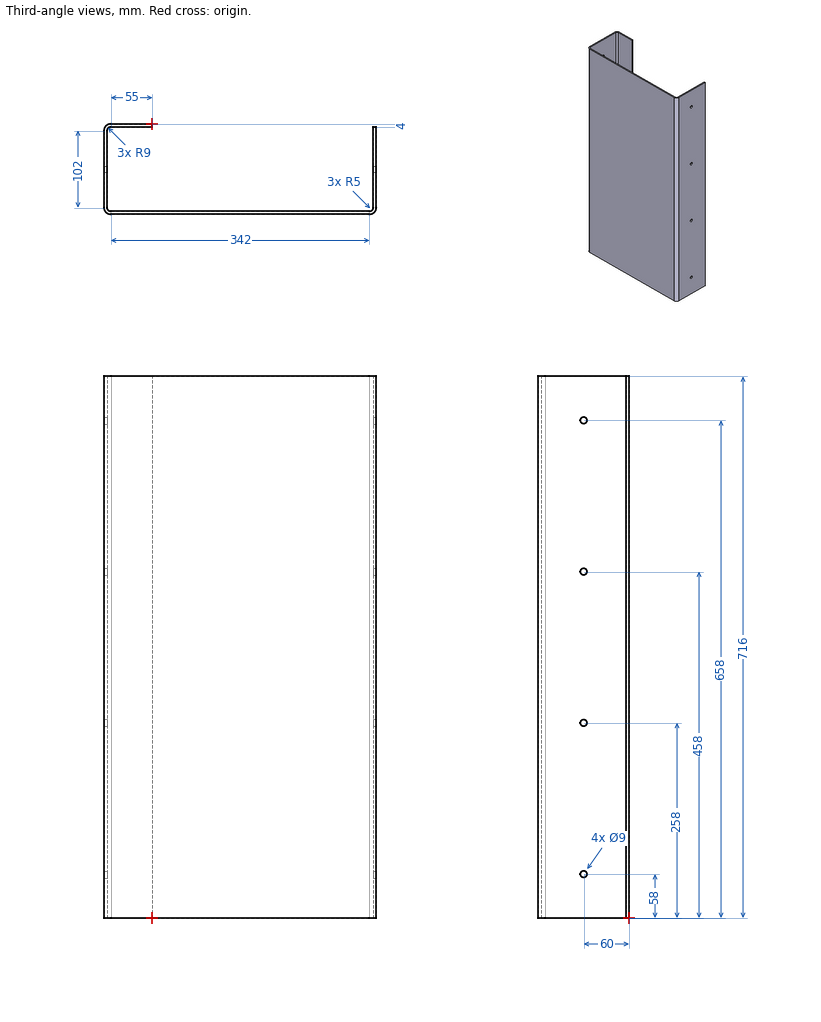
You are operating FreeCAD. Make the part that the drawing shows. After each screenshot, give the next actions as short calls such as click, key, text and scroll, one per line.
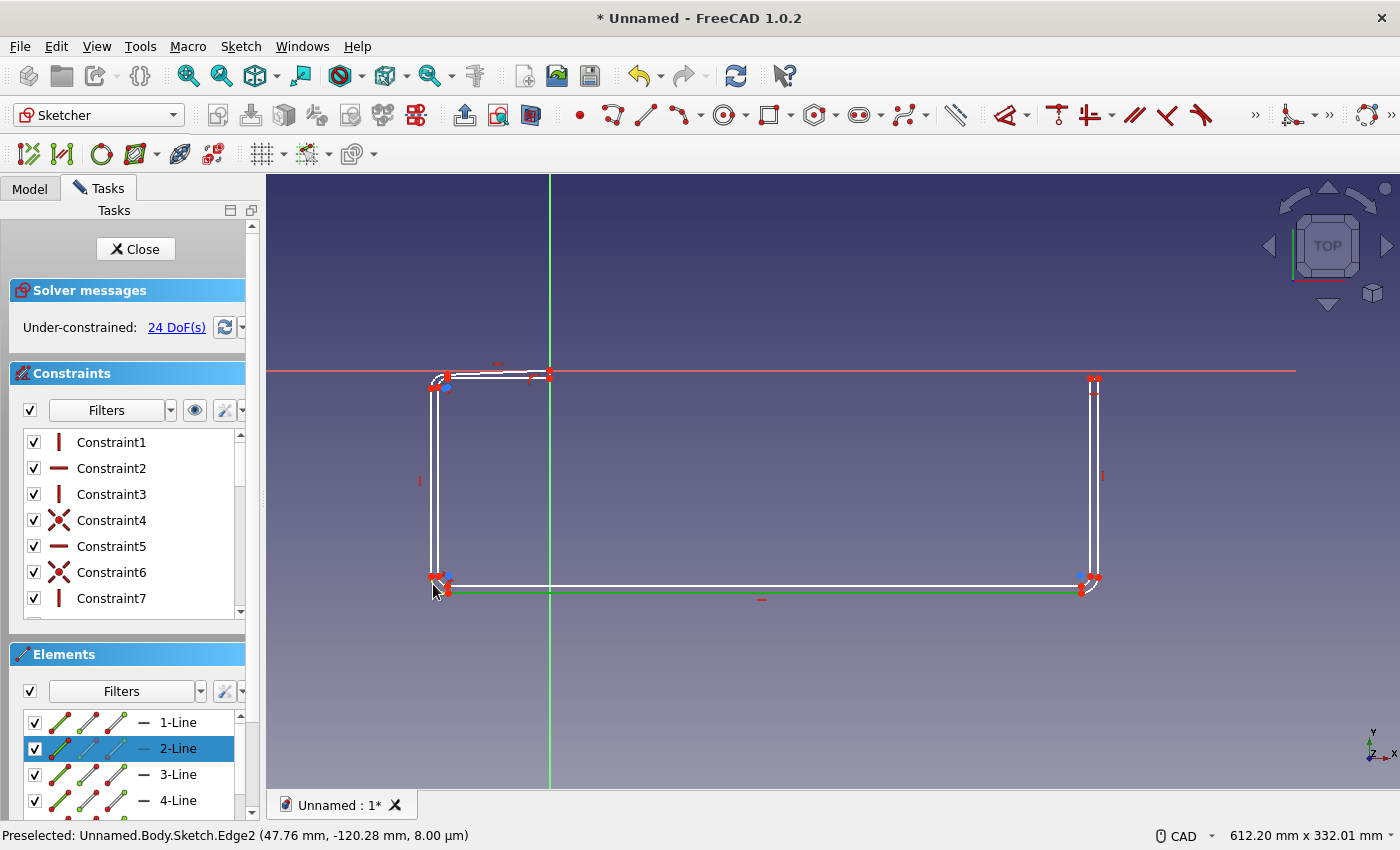
scroll(1088, 591, up, 4)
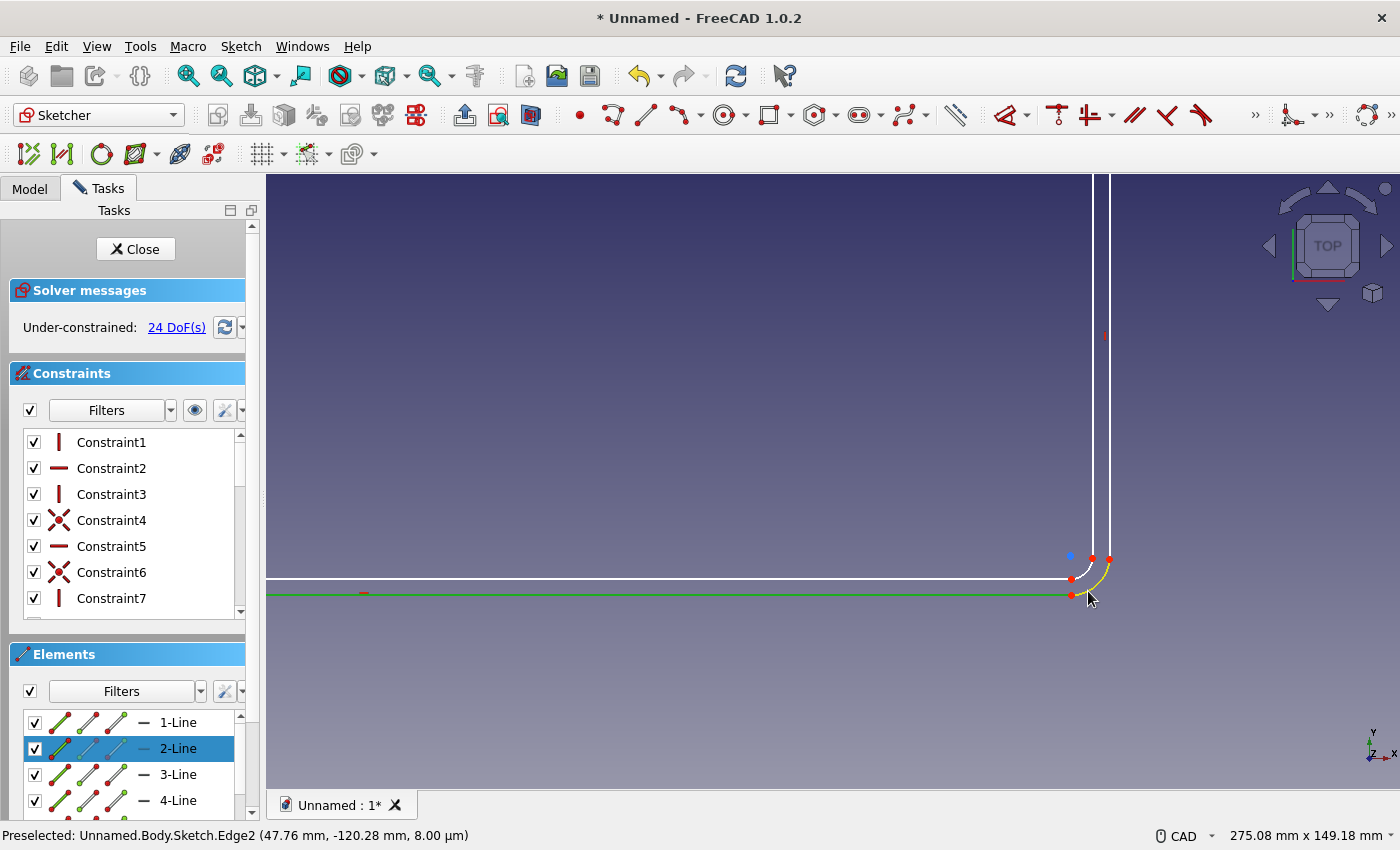
click(1088, 591)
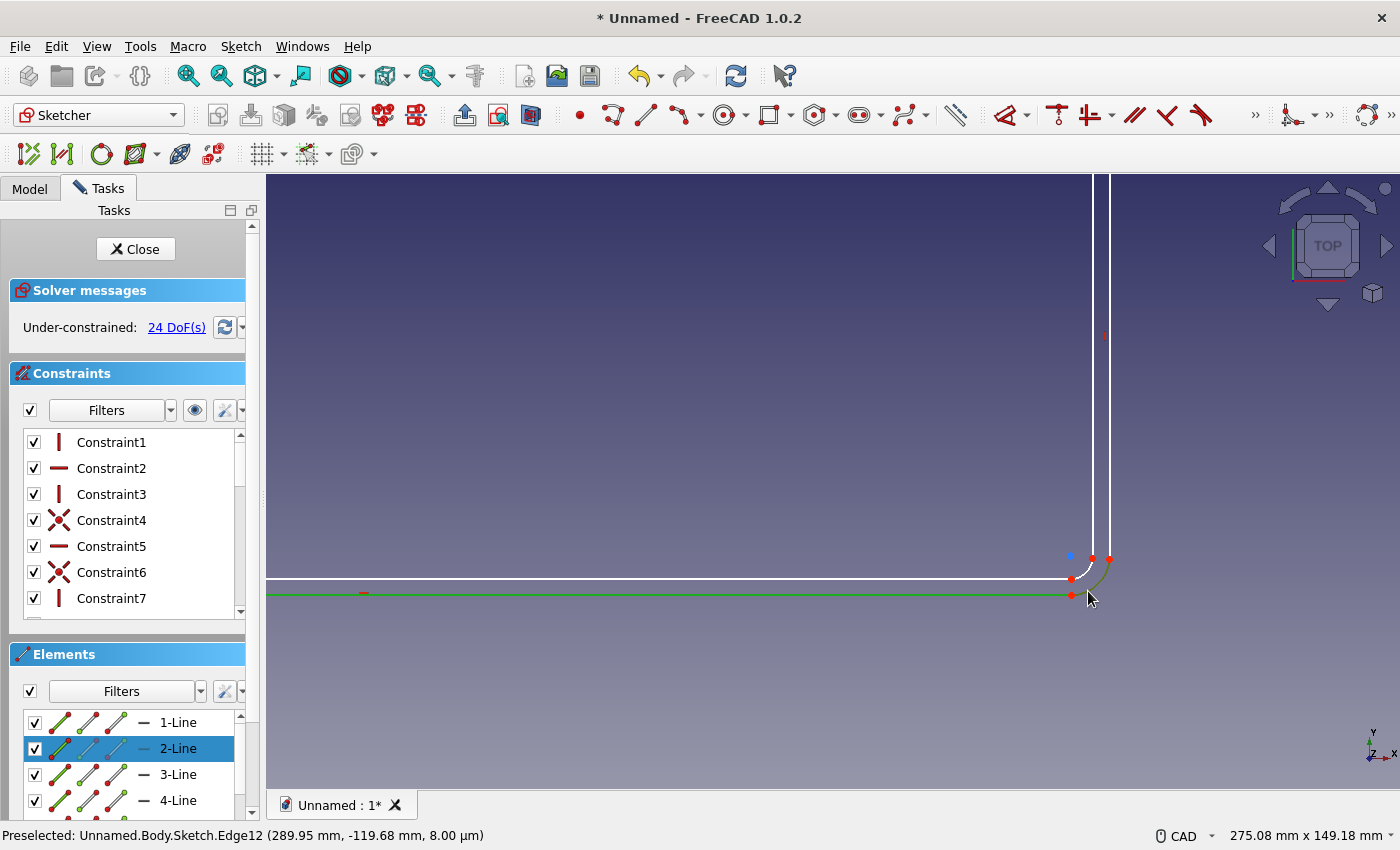
click(1201, 116)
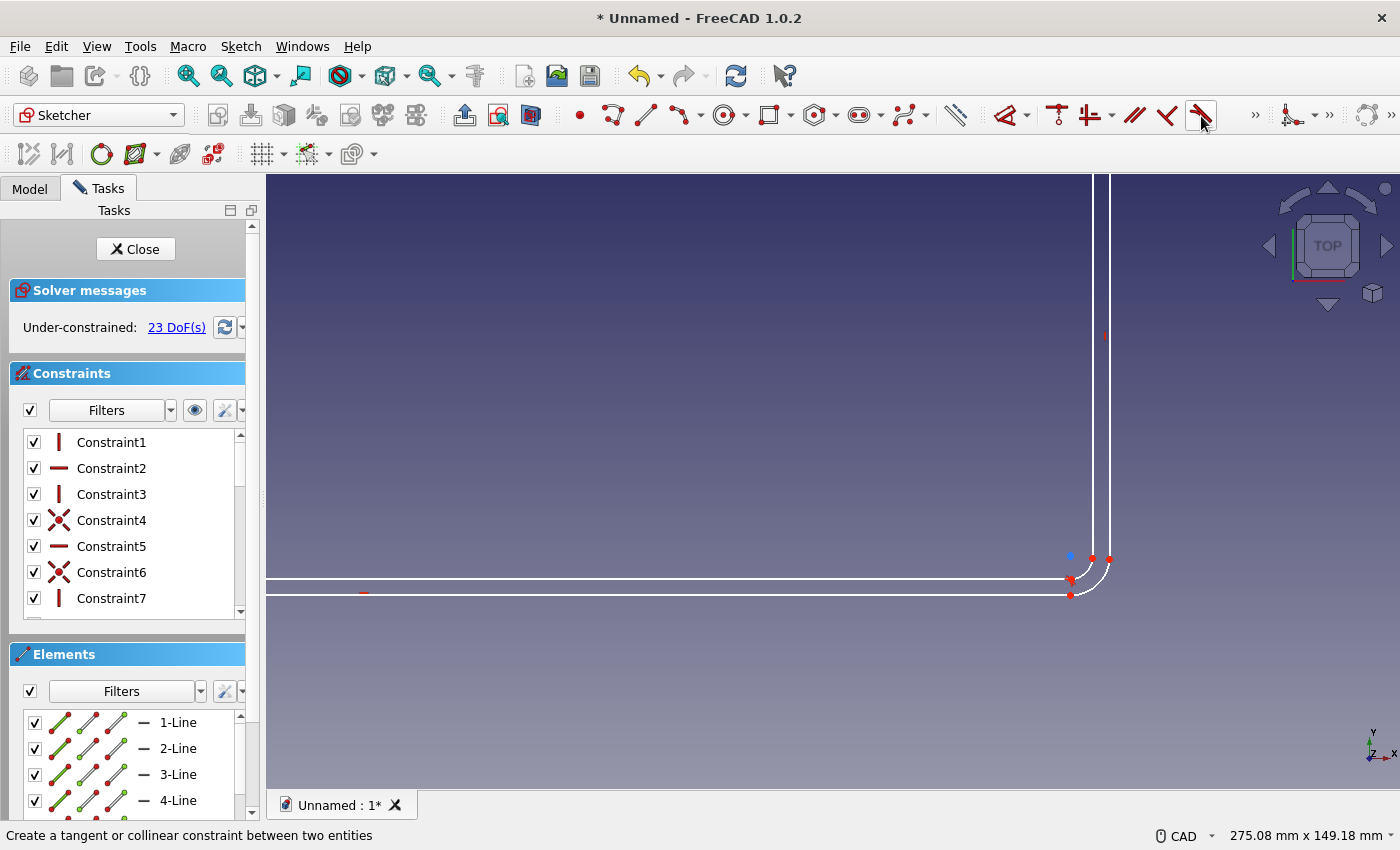
click(1110, 427)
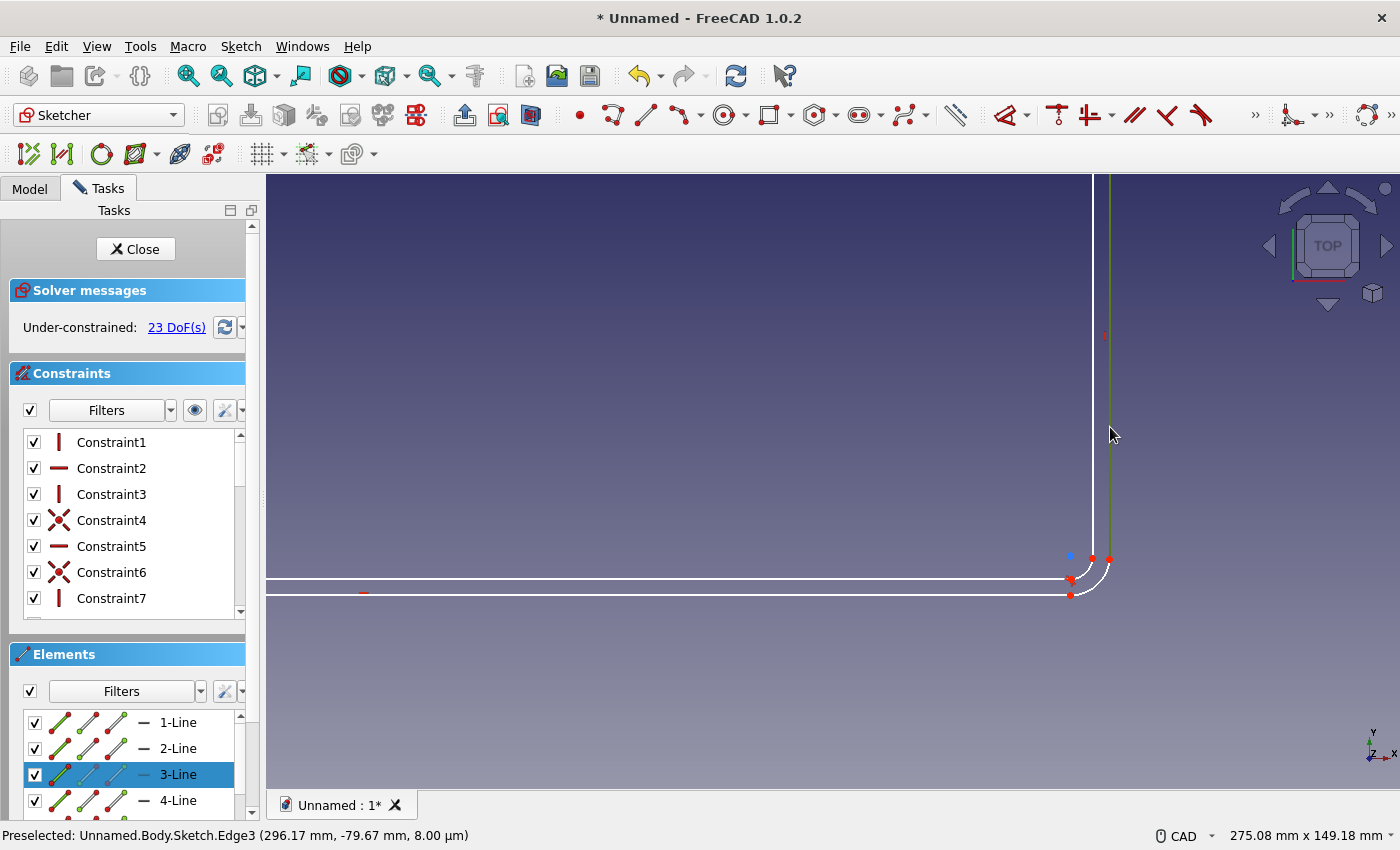
click(1087, 592)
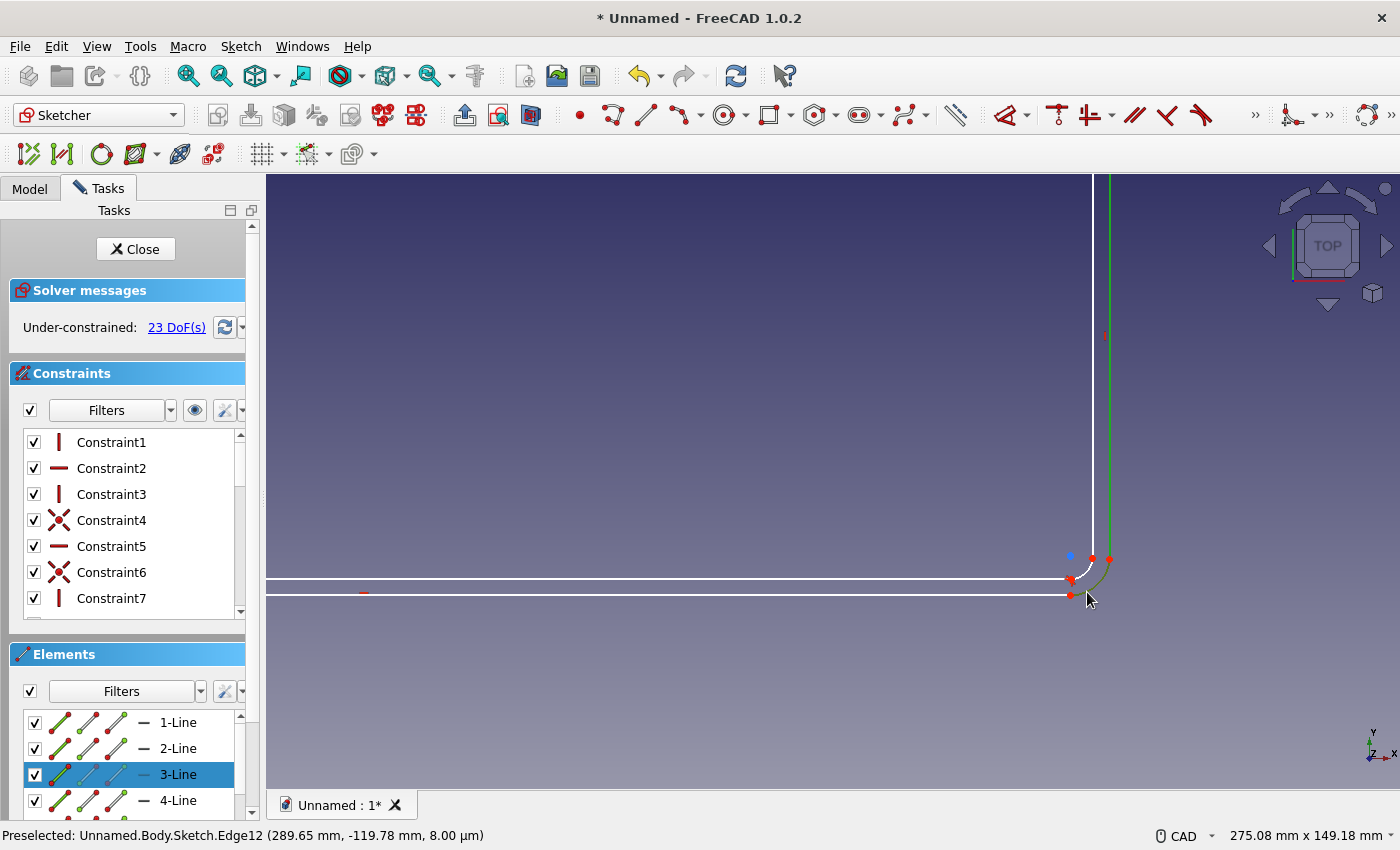
click(1201, 116)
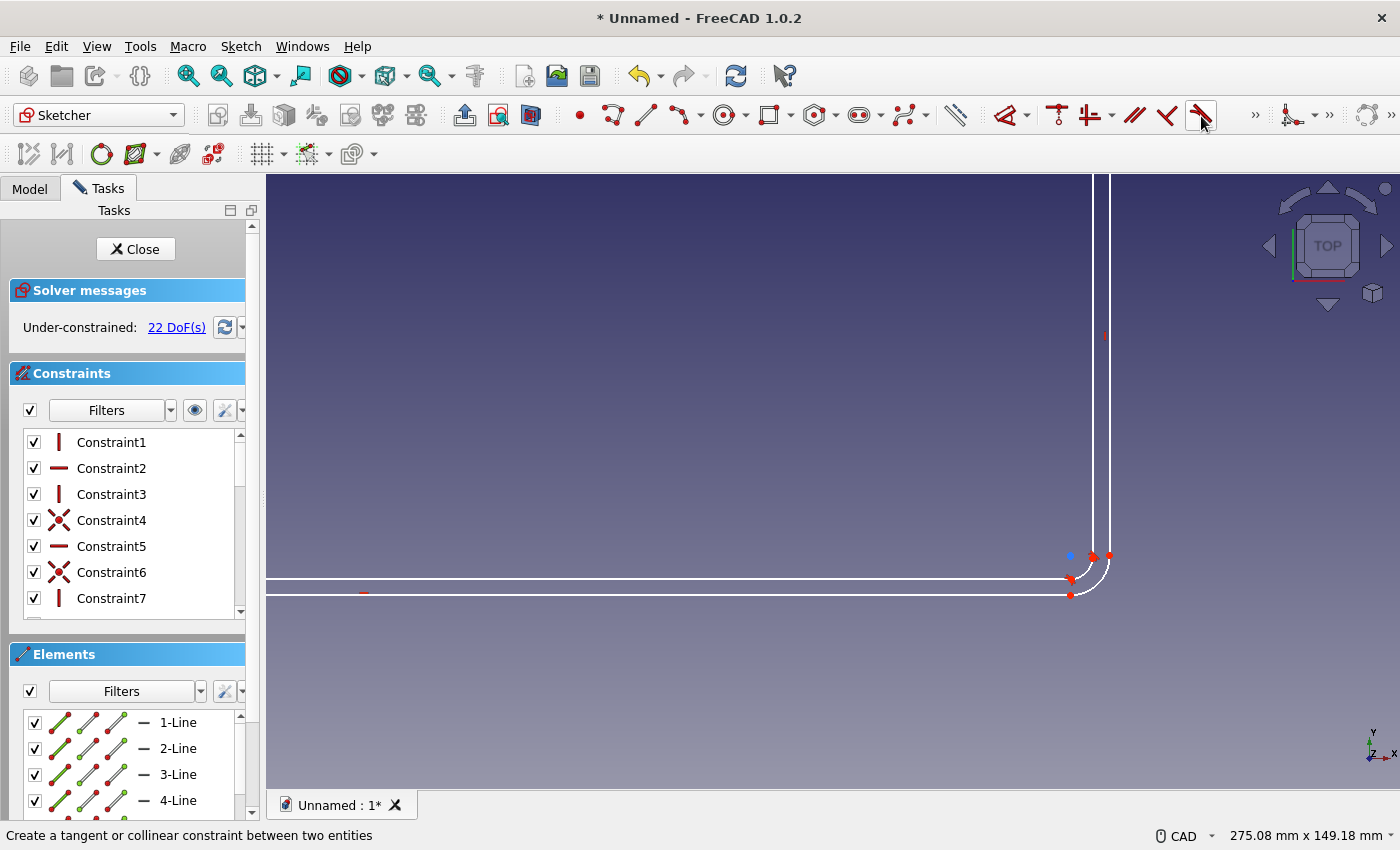
click(1093, 250)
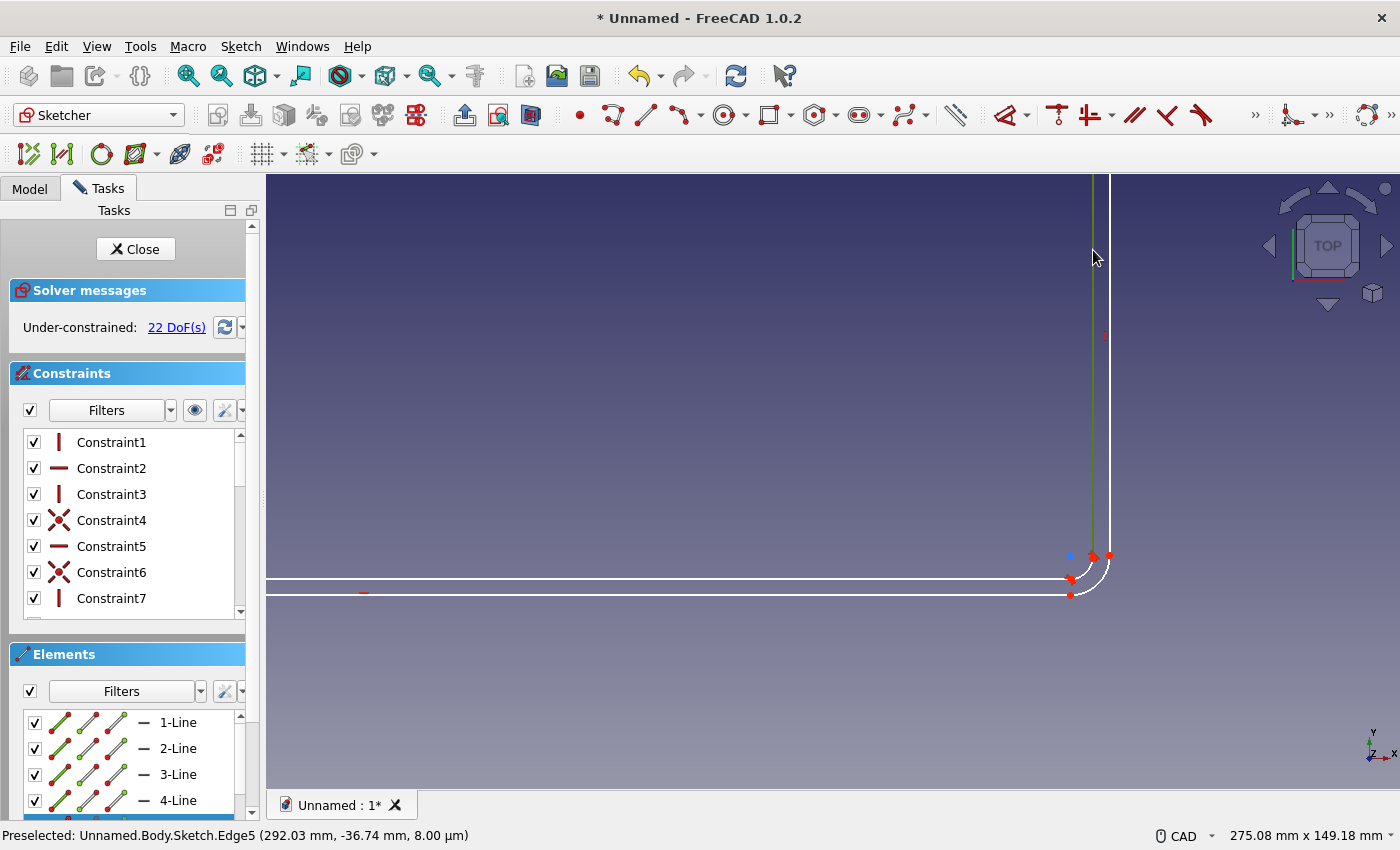
scroll(1081, 576, up, 2)